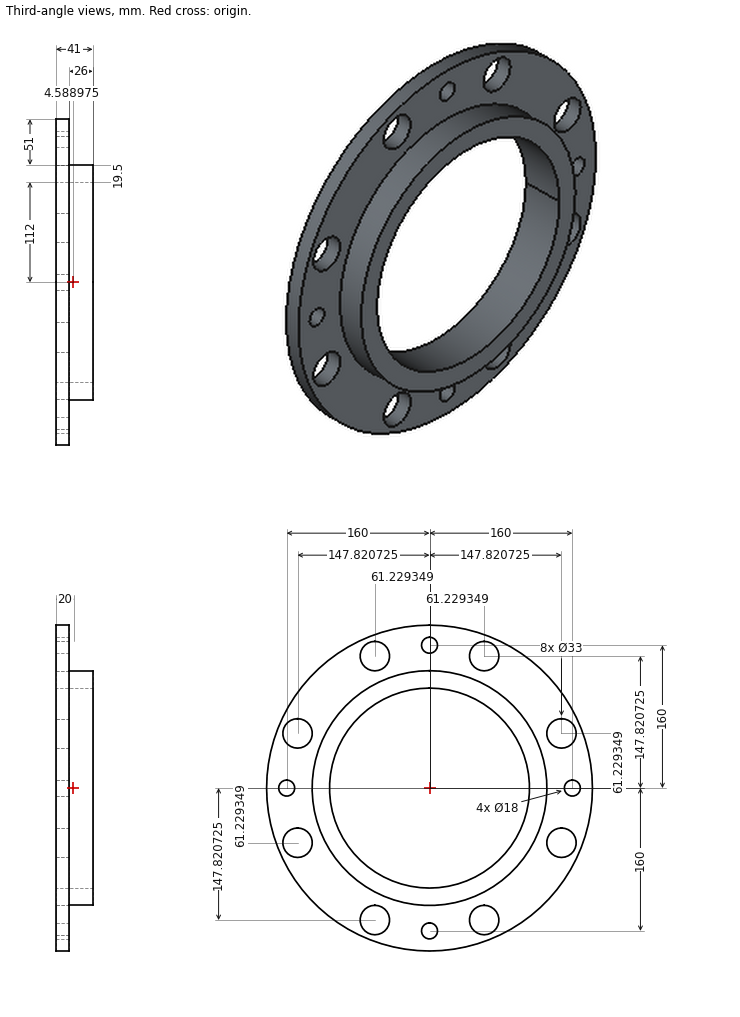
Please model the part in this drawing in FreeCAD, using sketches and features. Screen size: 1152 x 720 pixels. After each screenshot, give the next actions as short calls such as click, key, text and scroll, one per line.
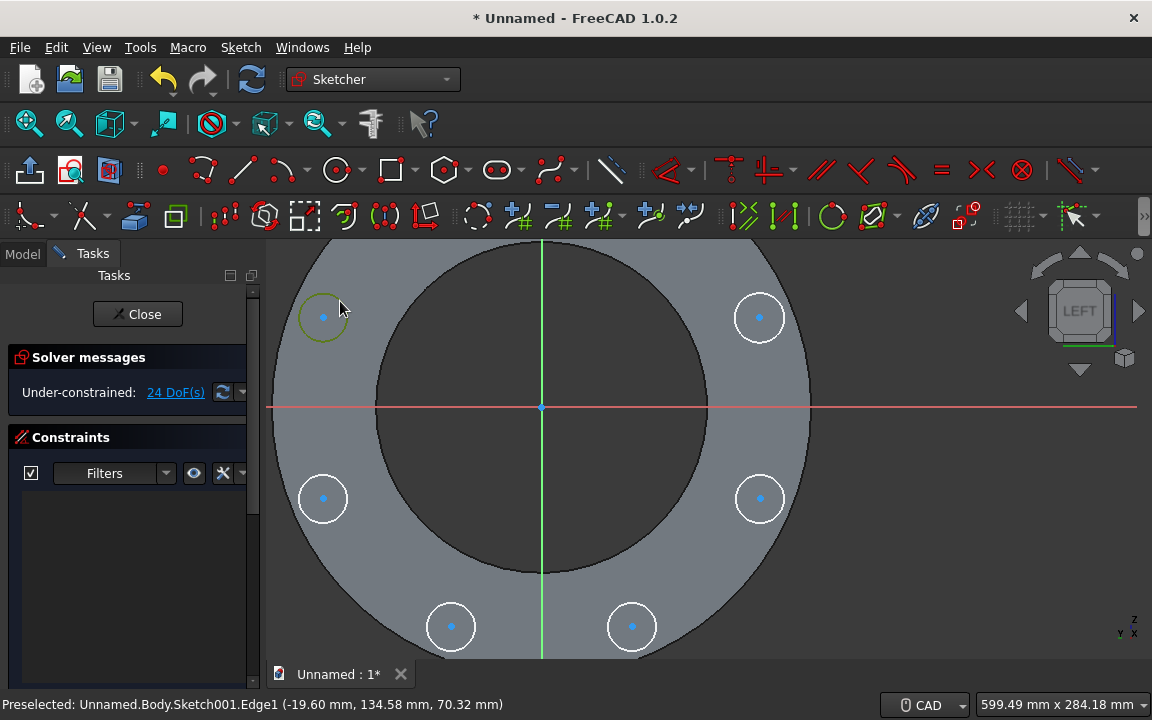
scroll(761, 500, down, 3)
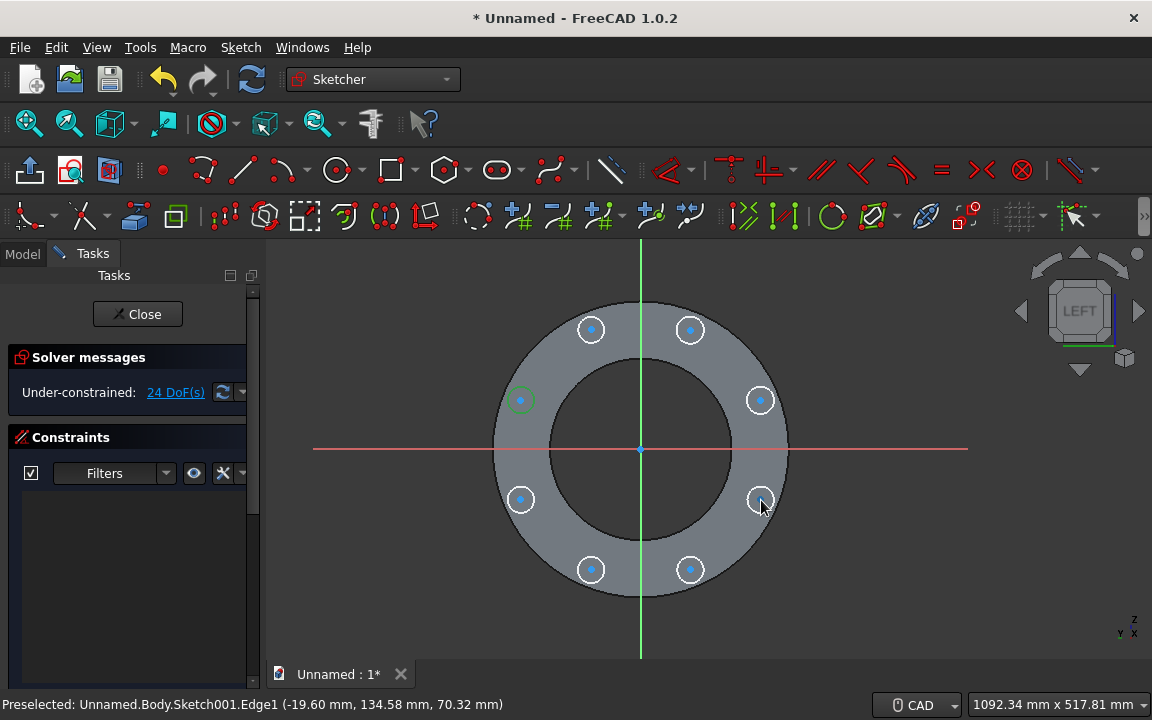
click(600, 321)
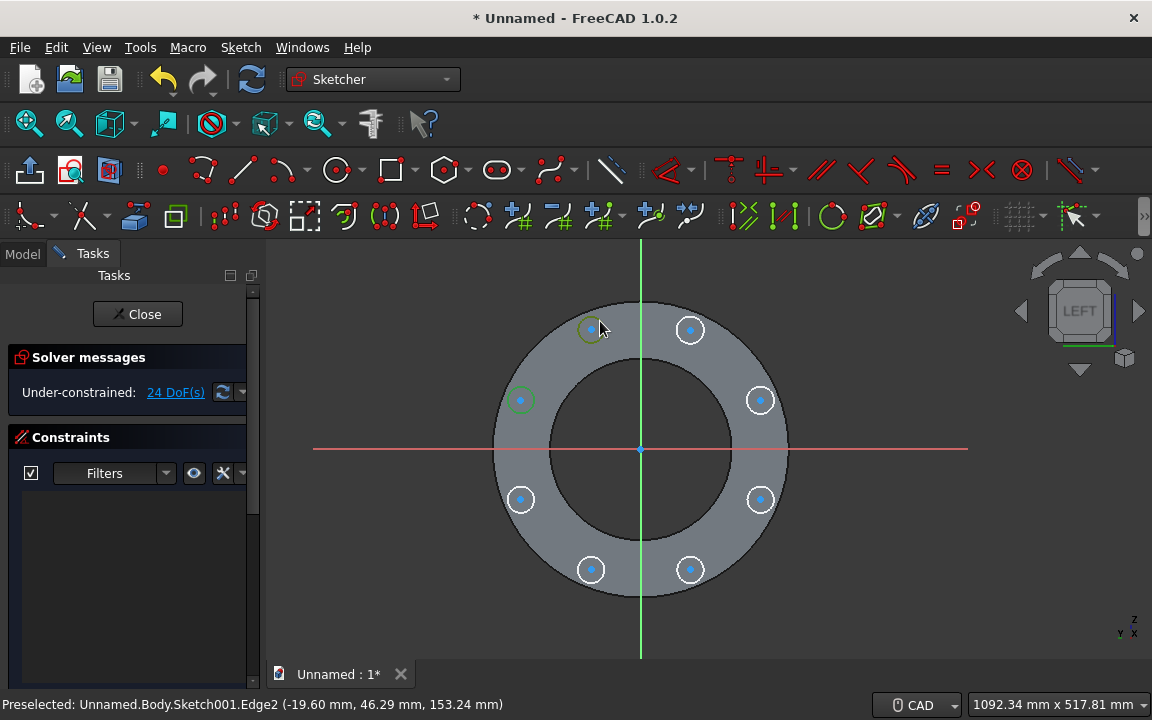
click(700, 320)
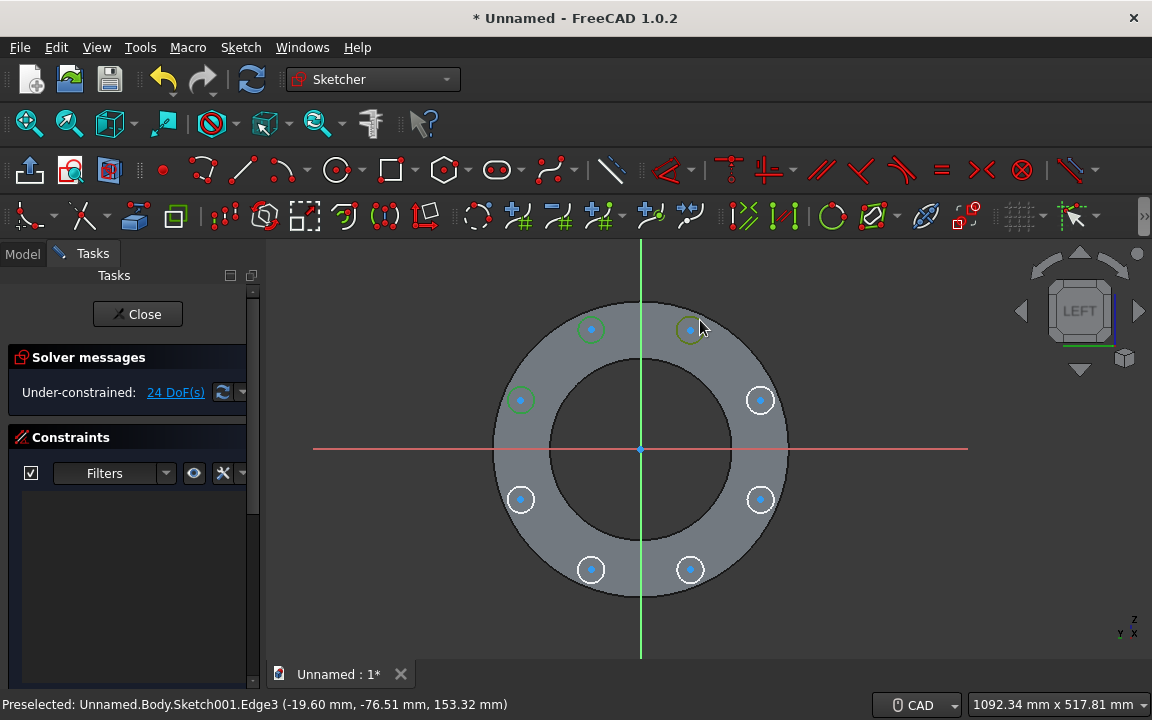
click(770, 391)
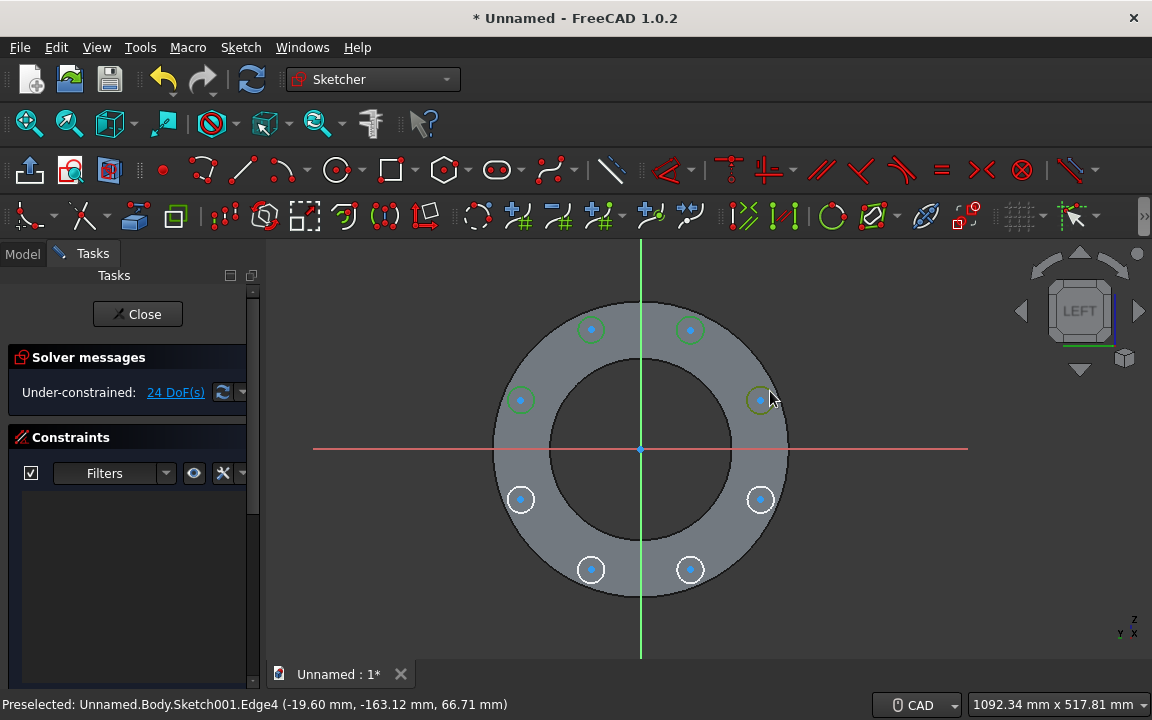
click(770, 490)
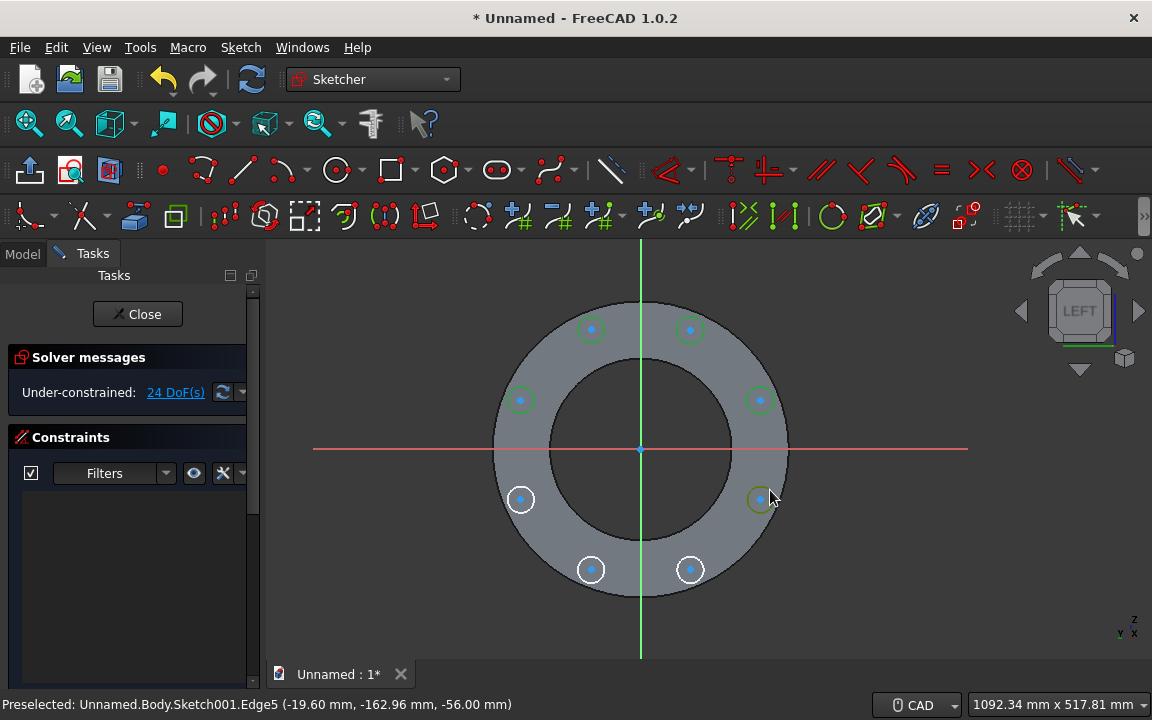
click(700, 561)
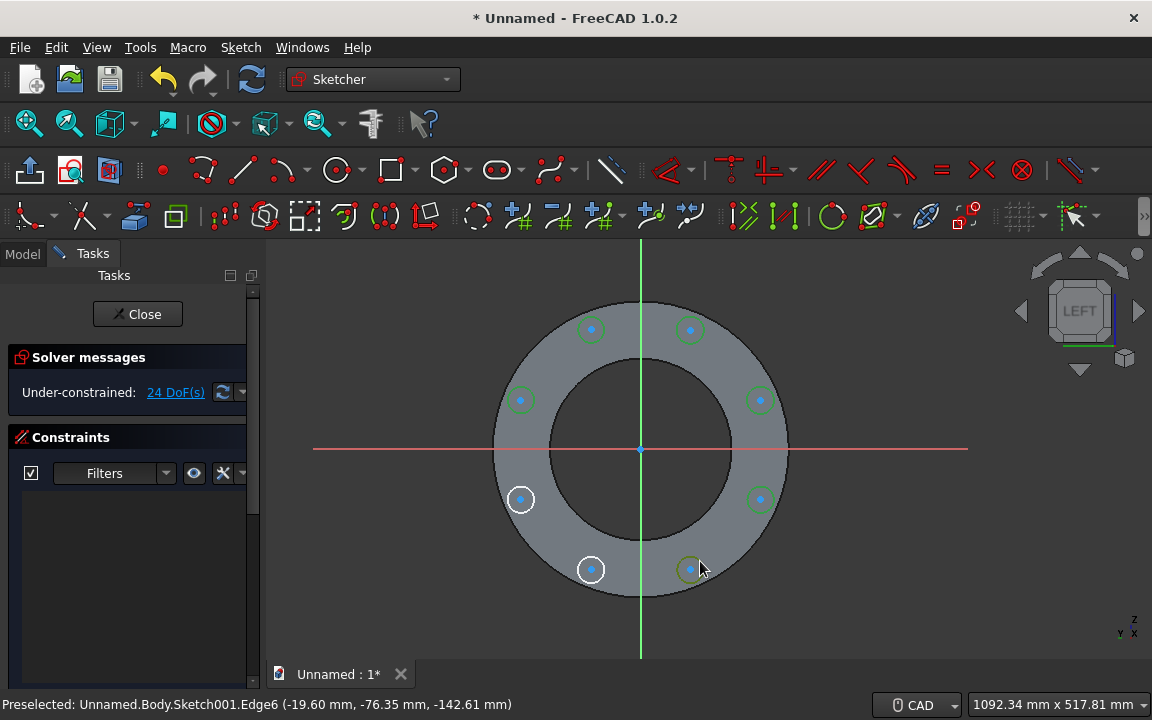
click(600, 561)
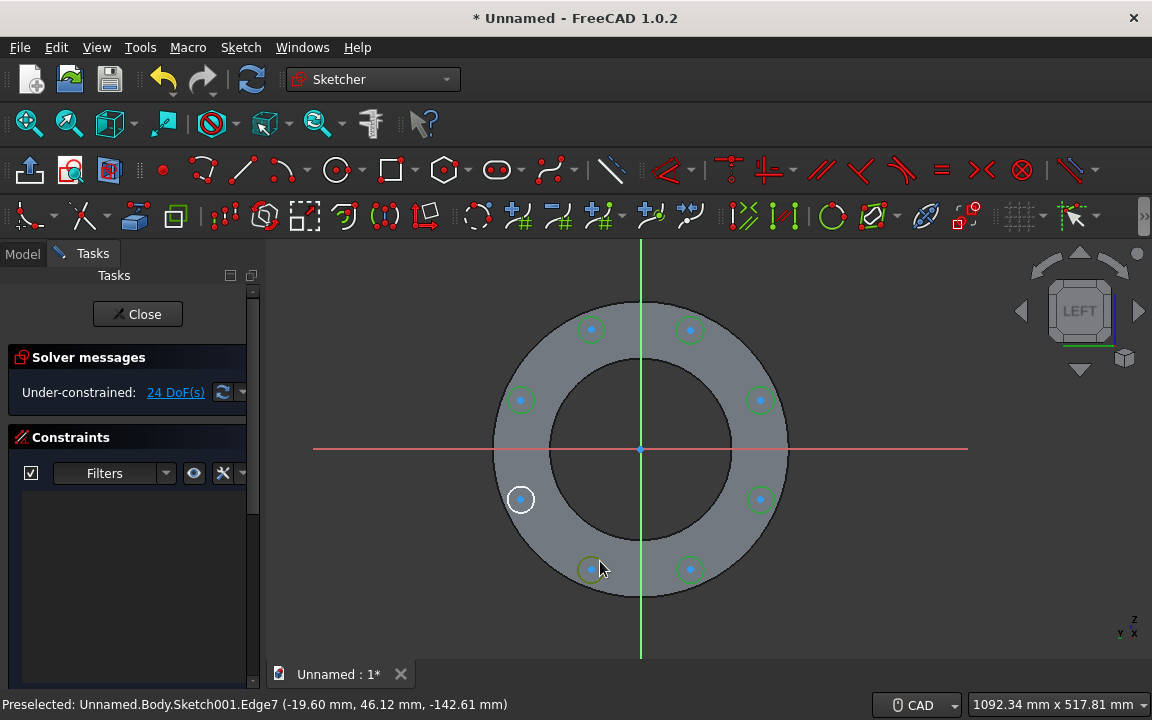
click(530, 490)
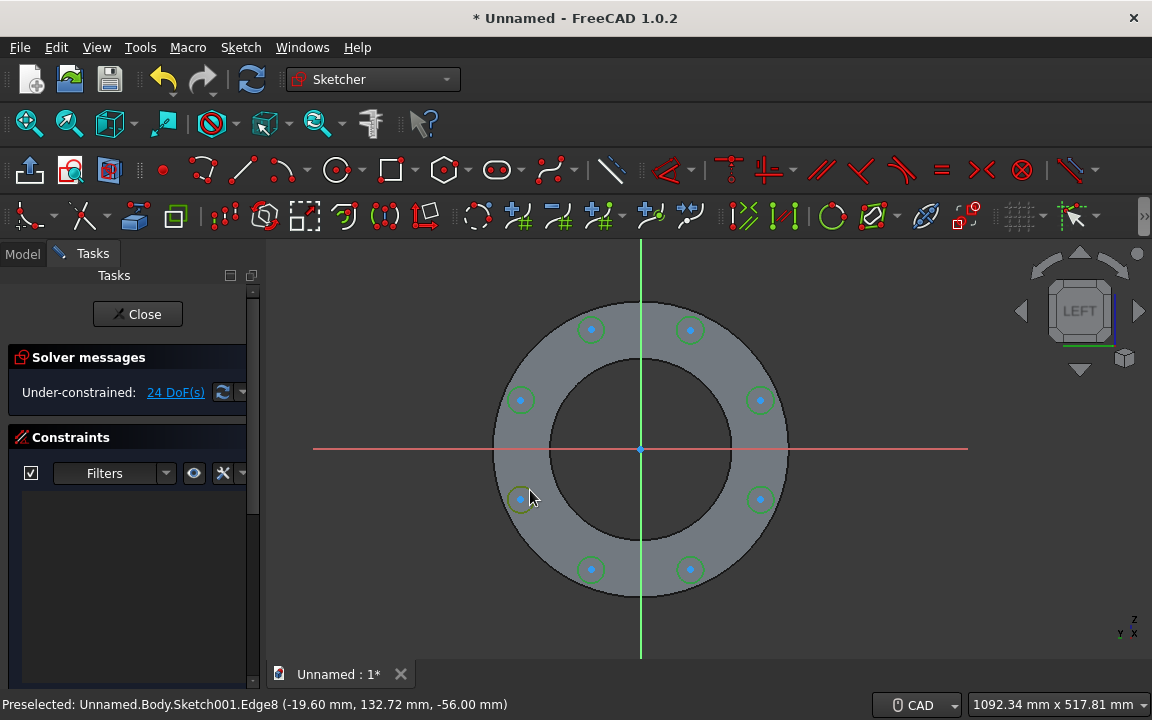
click(942, 170)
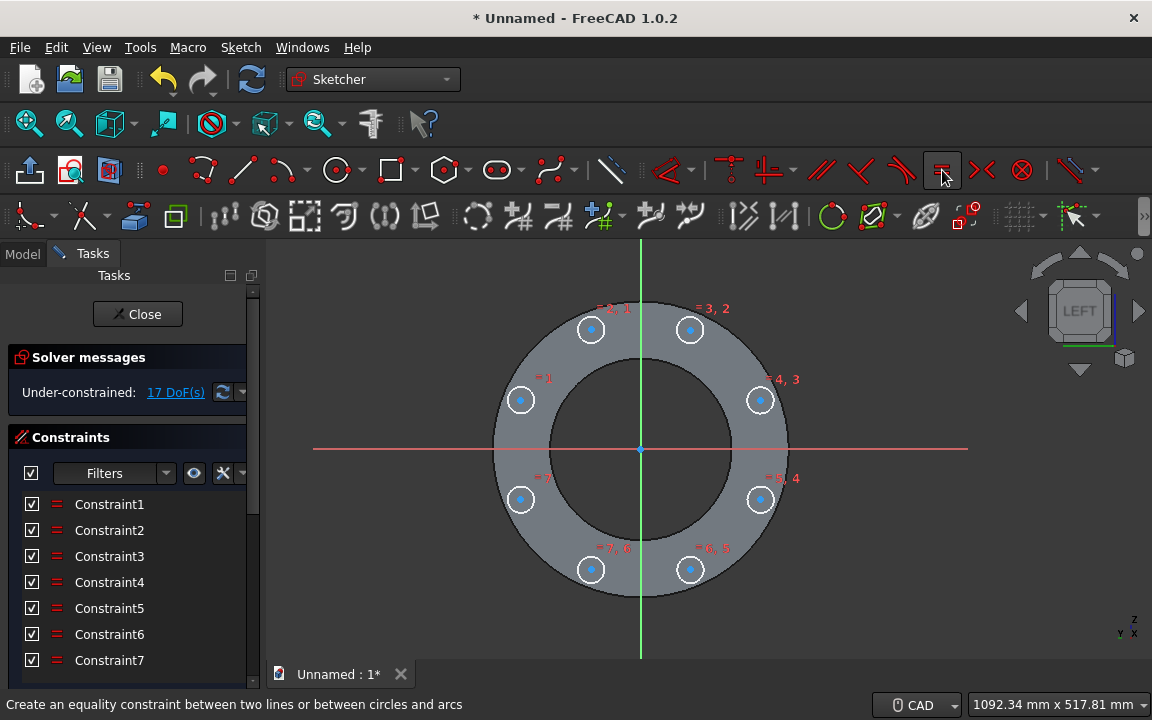
click(591, 330)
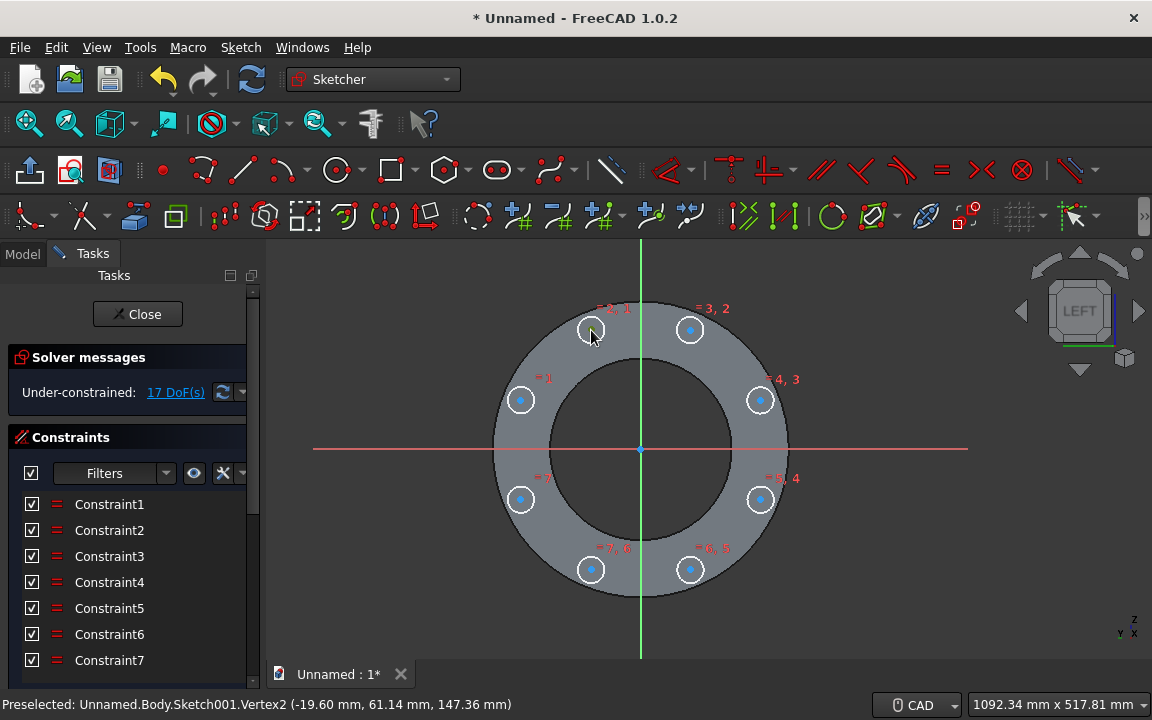
click(690, 330)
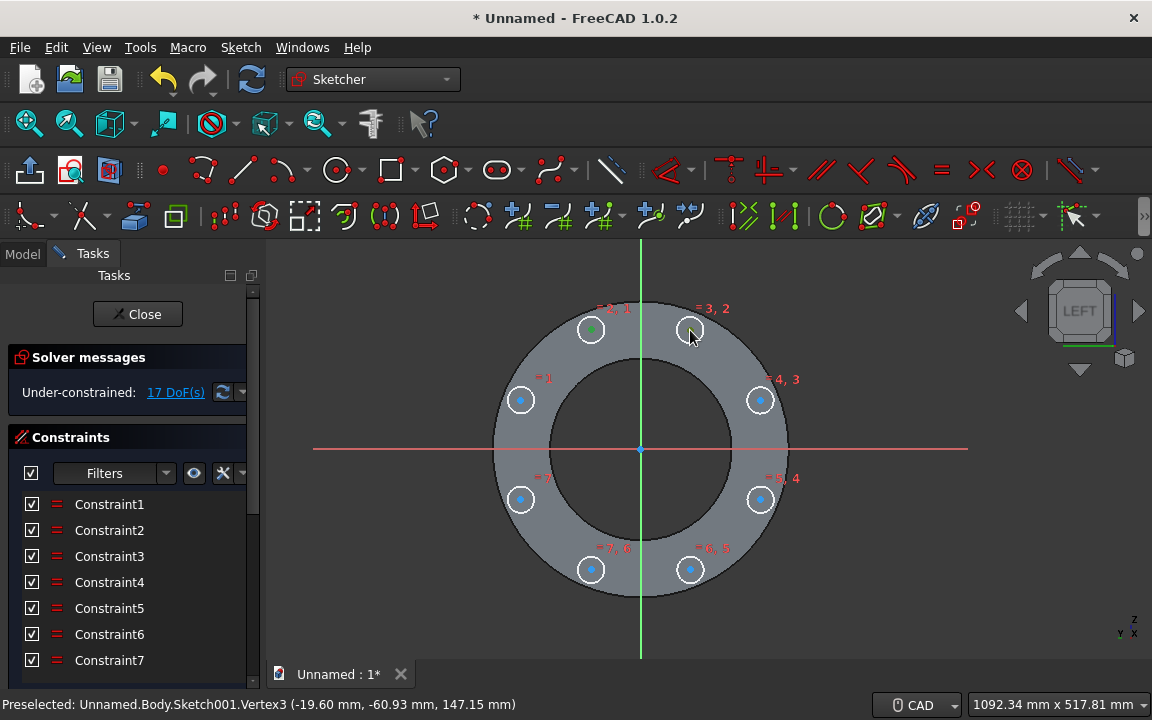
key(h)